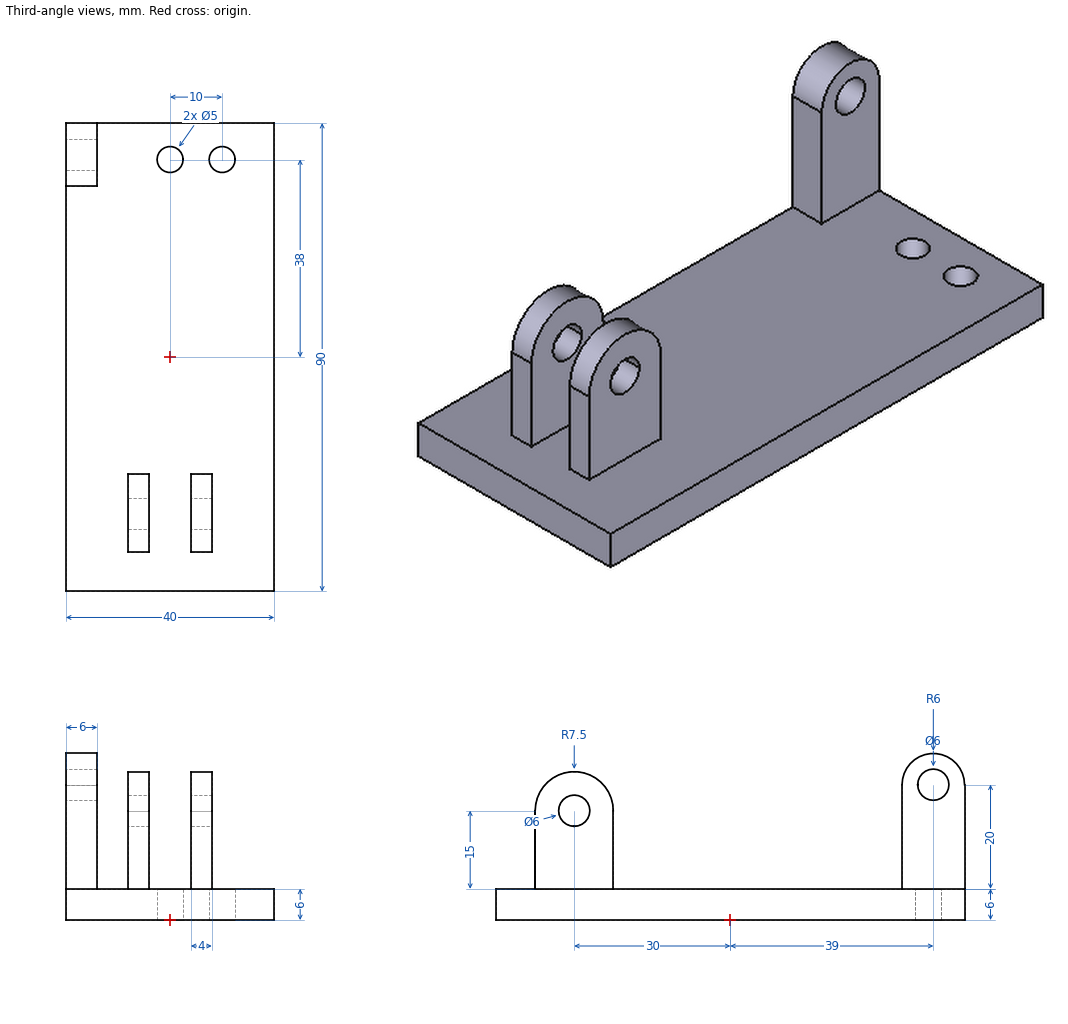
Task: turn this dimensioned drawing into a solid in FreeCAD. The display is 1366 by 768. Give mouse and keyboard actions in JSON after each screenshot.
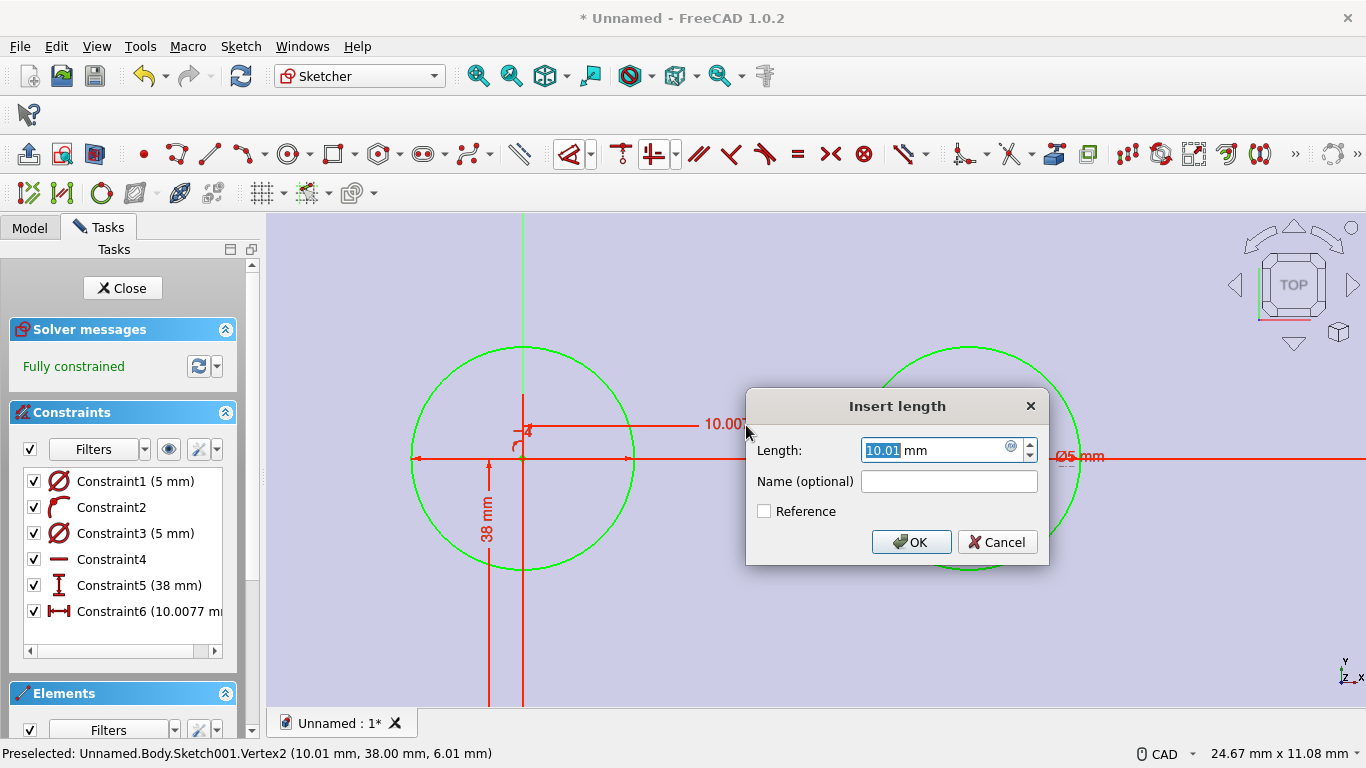
{"action": "type", "text": "10"}
{"action": "key", "text": "Return"}
{"action": "key", "text": "Escape"}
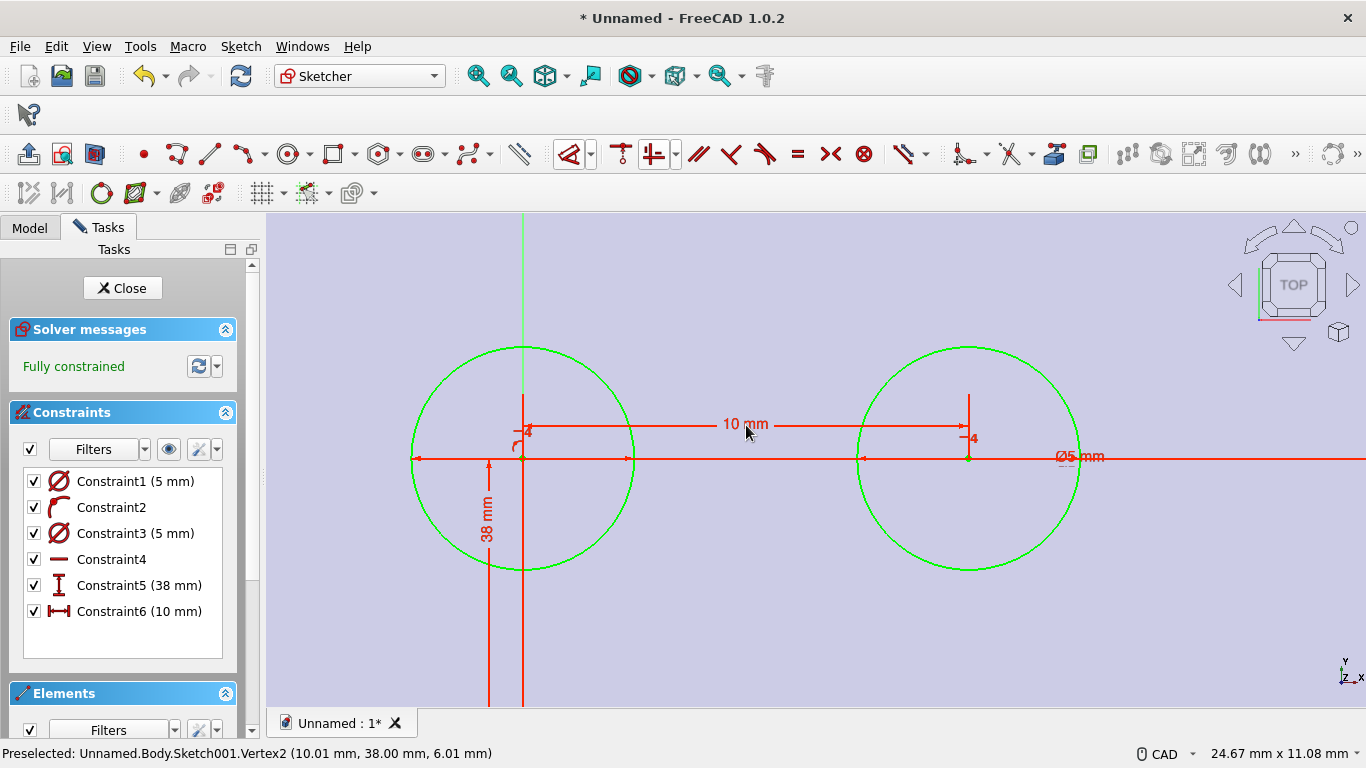
{"action": "left_click", "coordinate": [123, 288]}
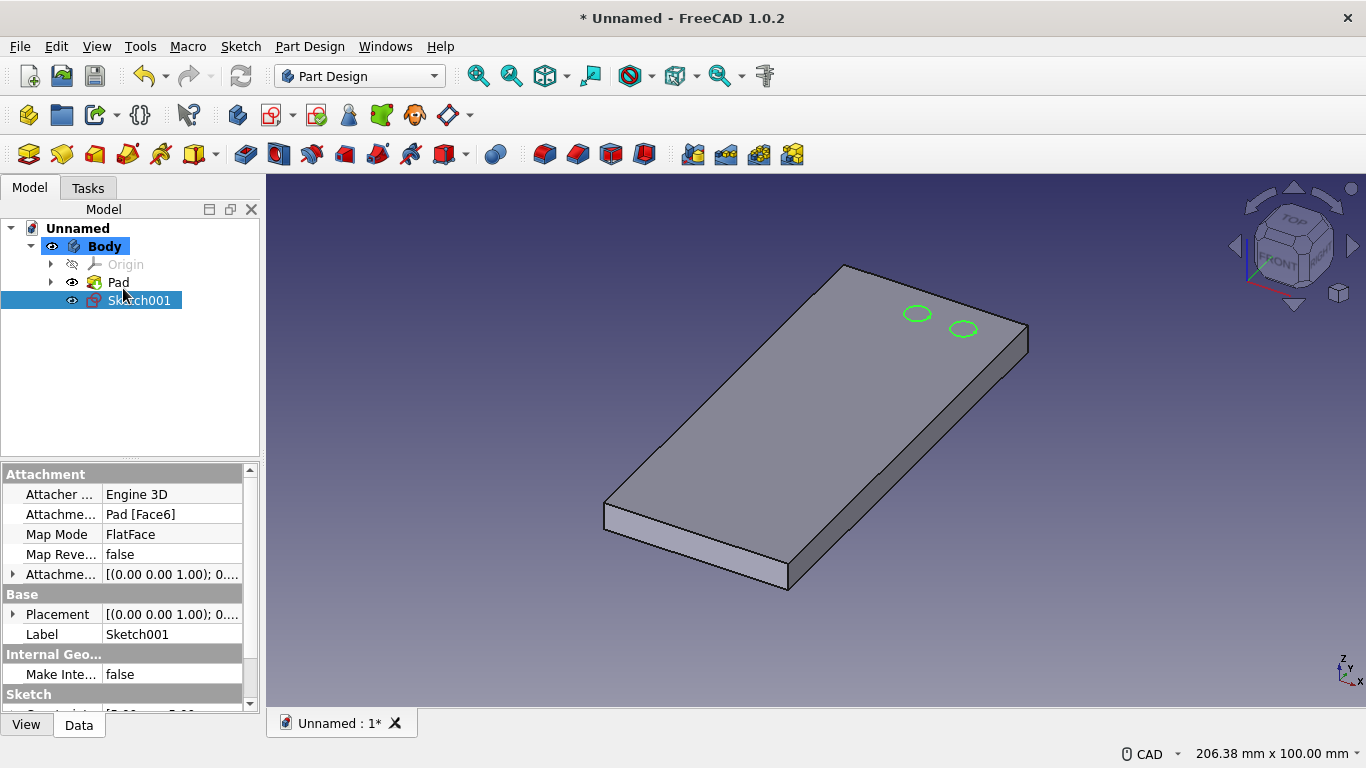
{"action": "left_click", "coordinate": [246, 154]}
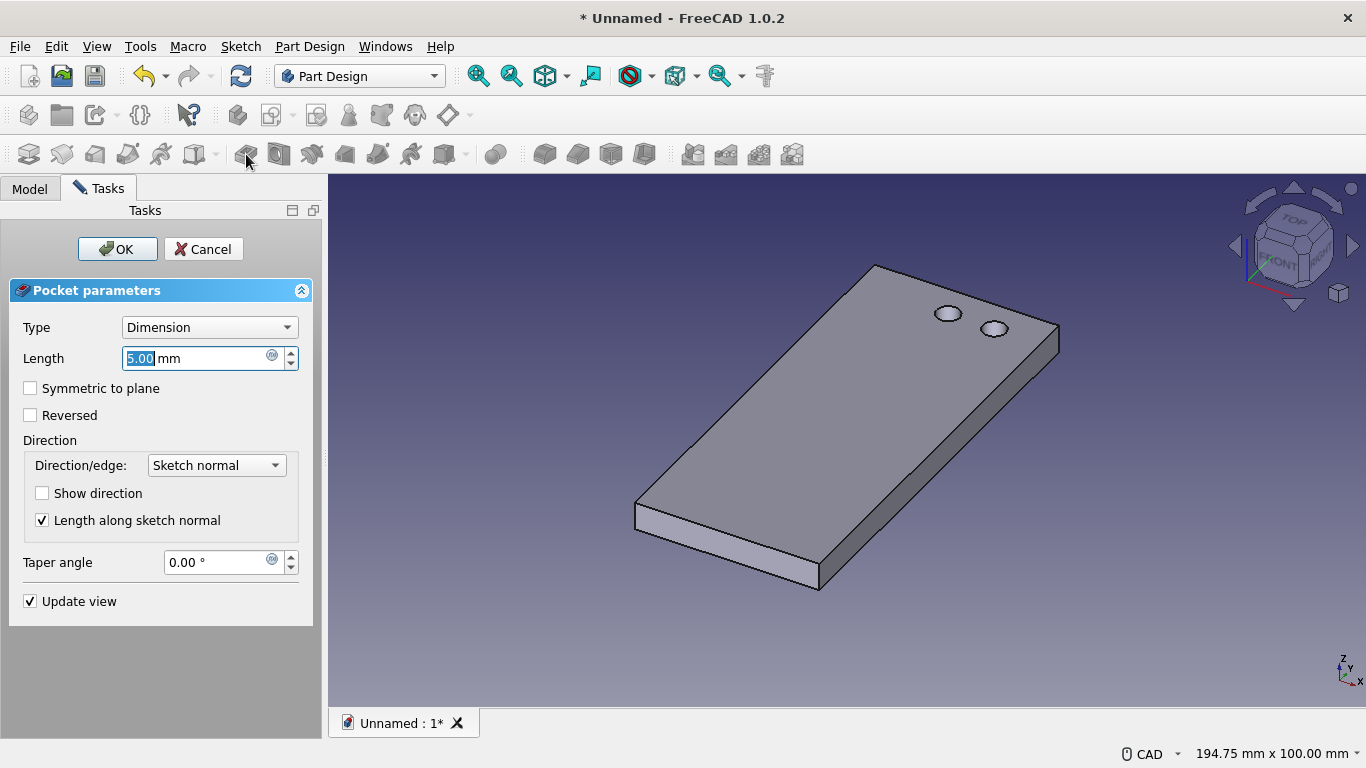
{"action": "type", "text": "6"}
{"action": "key", "text": "Tab"}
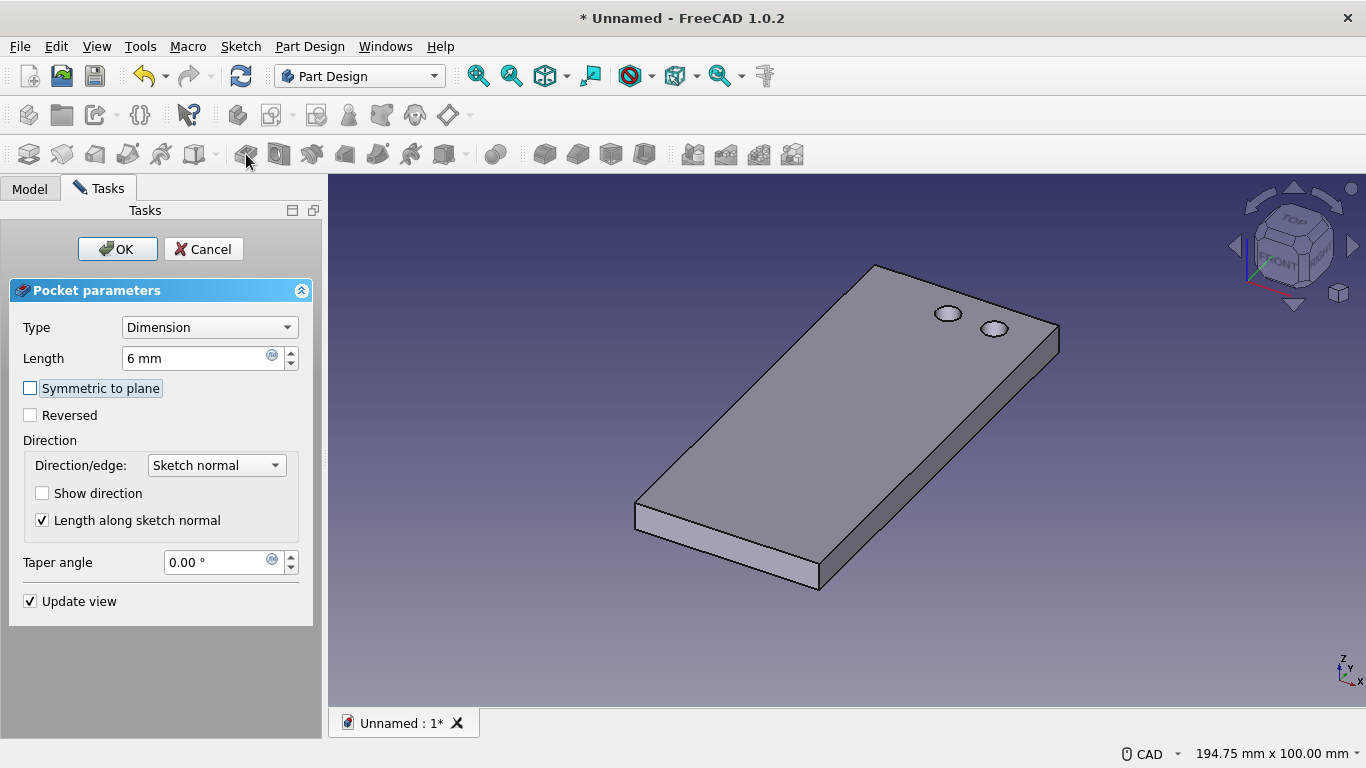
{"action": "left_click", "coordinate": [118, 249]}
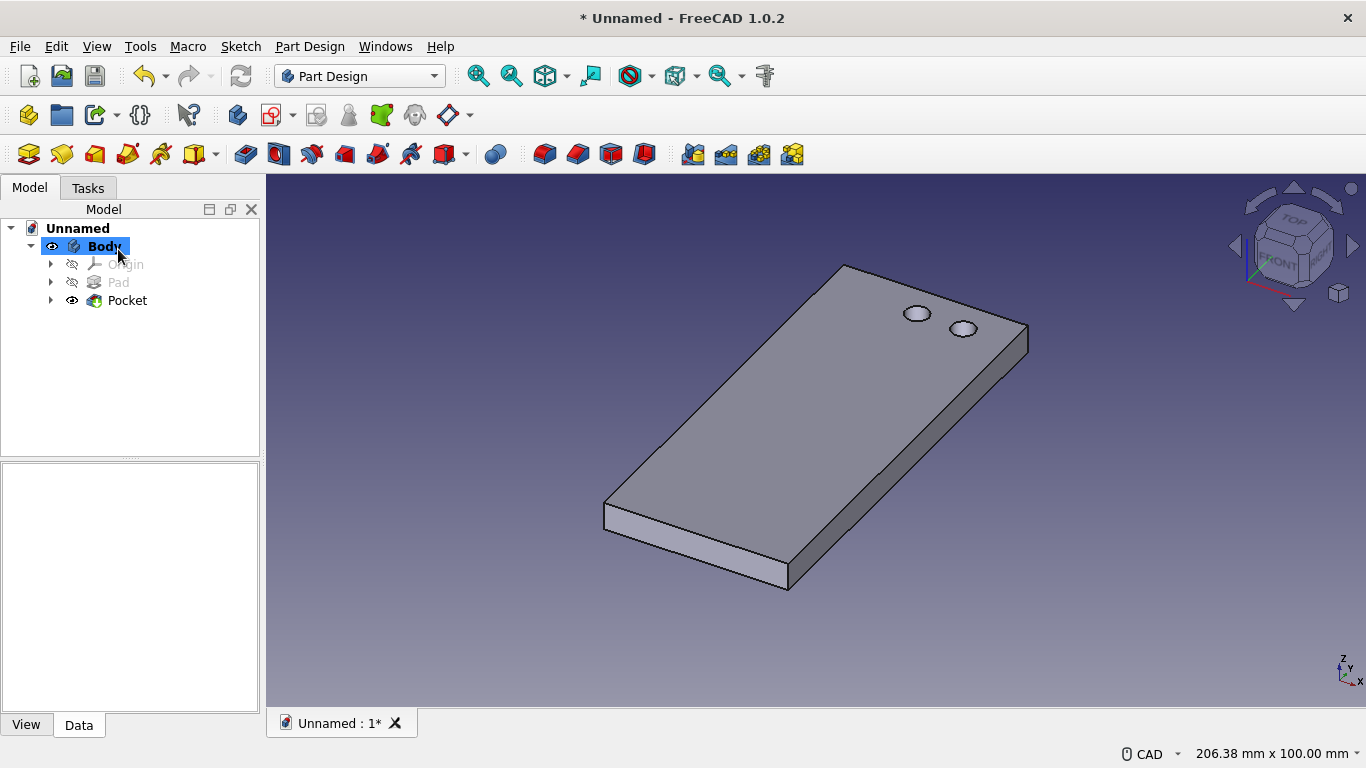
{"action": "key", "text": "6"}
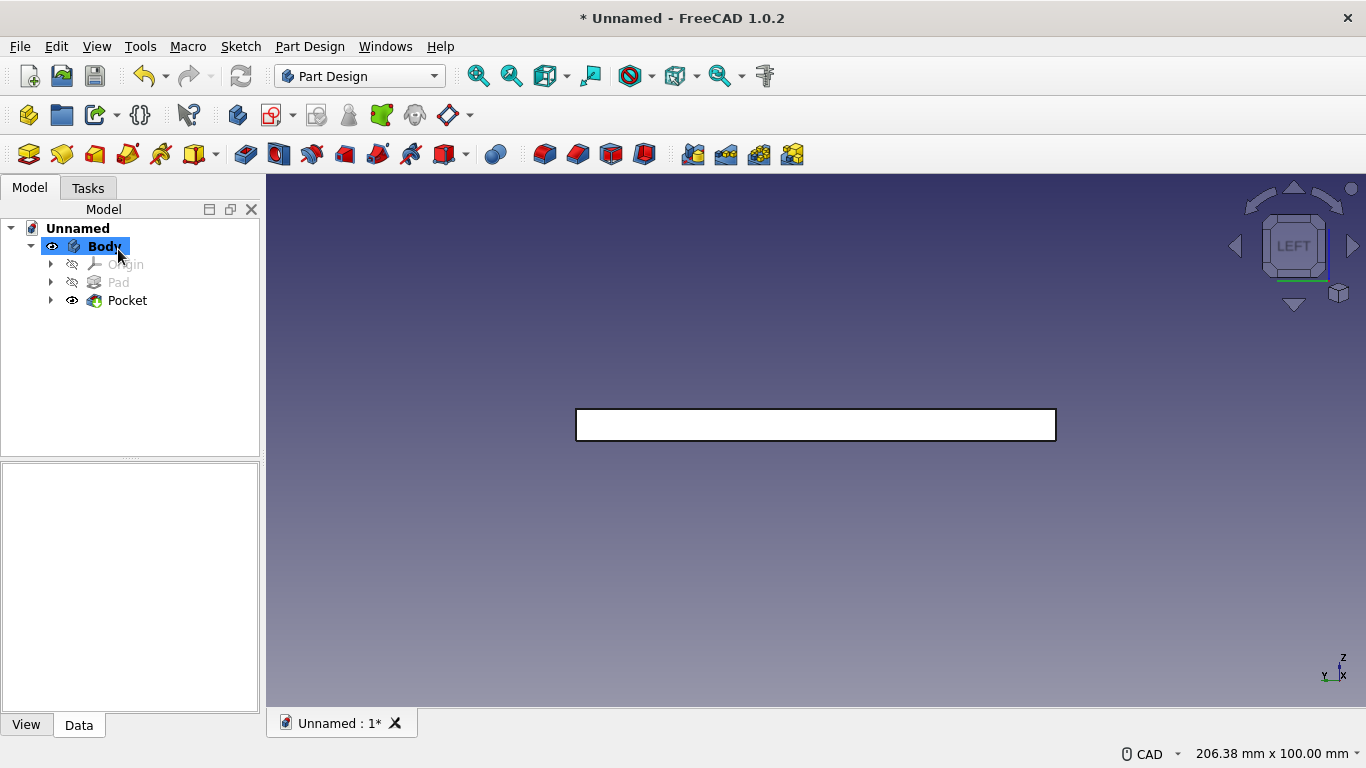
{"action": "left_click", "coordinate": [479, 76]}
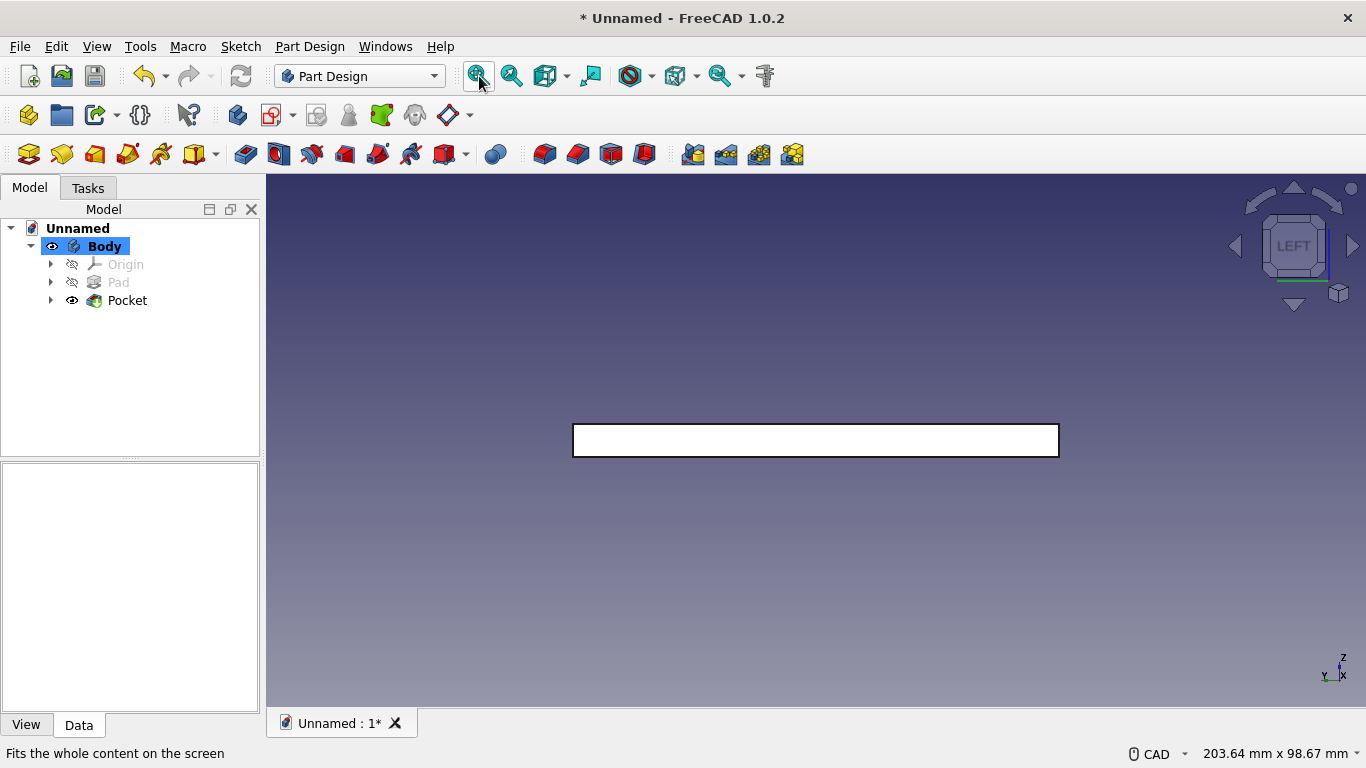
{"action": "left_click", "coordinate": [608, 439]}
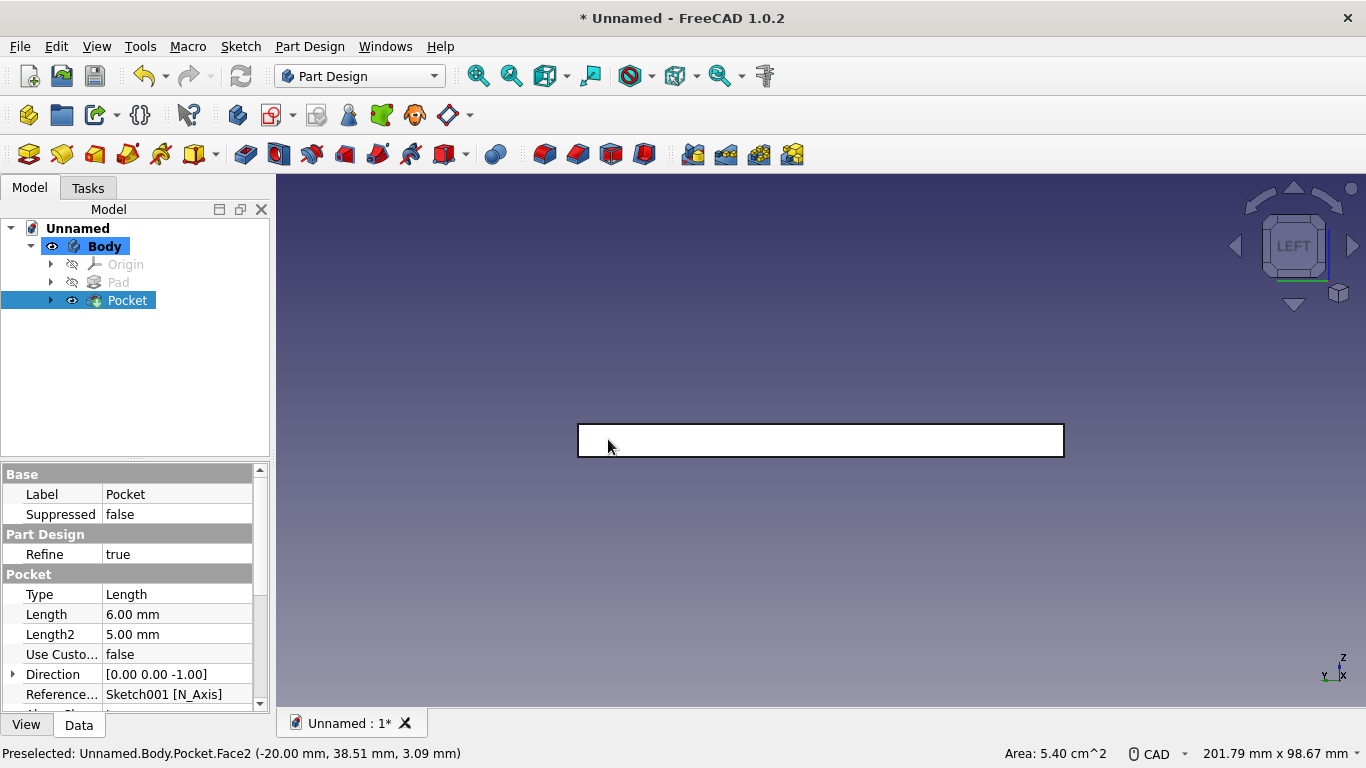
{"action": "left_click", "coordinate": [270, 116]}